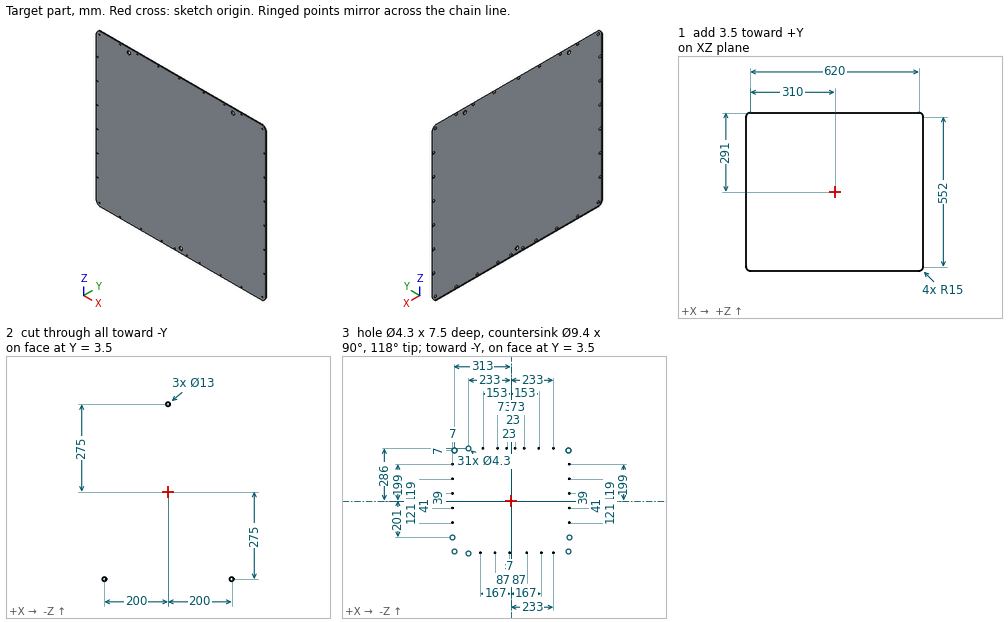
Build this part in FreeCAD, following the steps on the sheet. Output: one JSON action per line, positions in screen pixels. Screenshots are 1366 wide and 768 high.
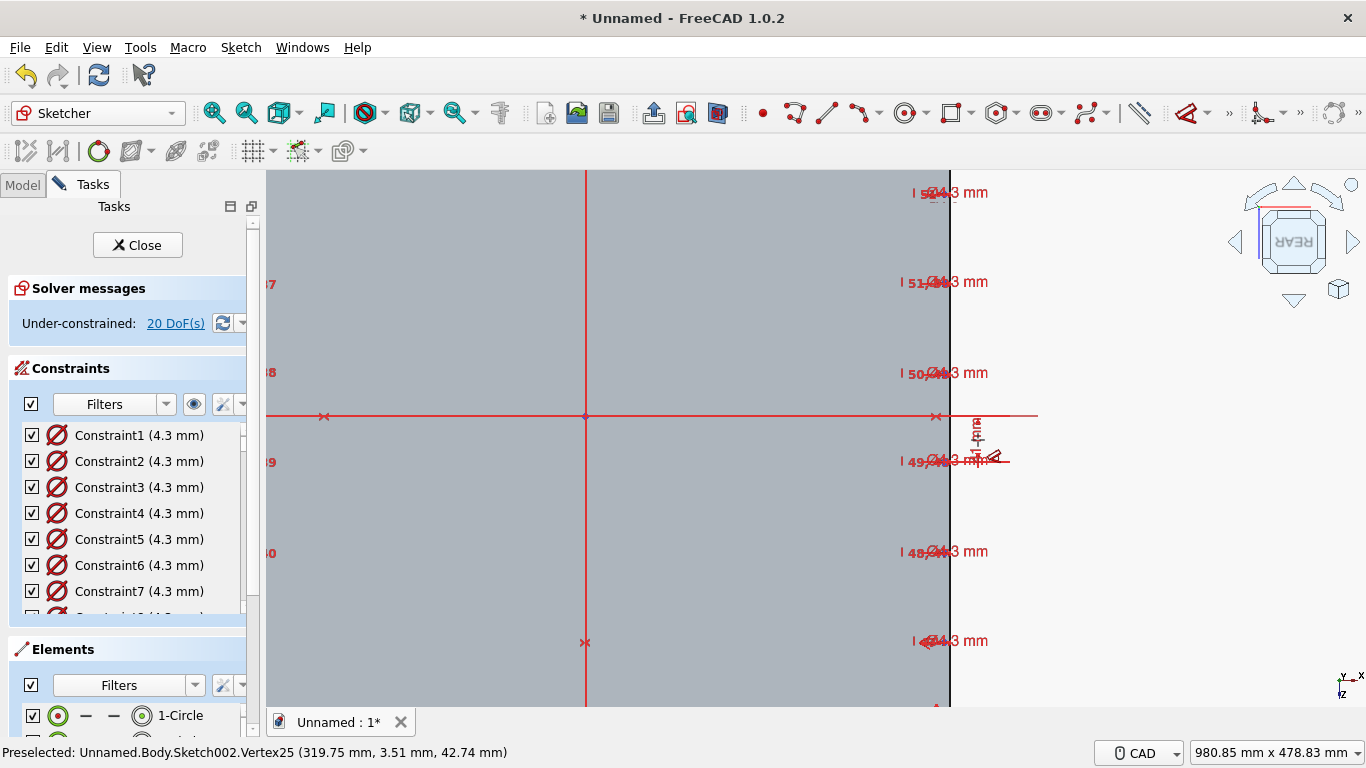
{"action": "left_click", "coordinate": [944, 375]}
{"action": "left_click", "coordinate": [978, 396]}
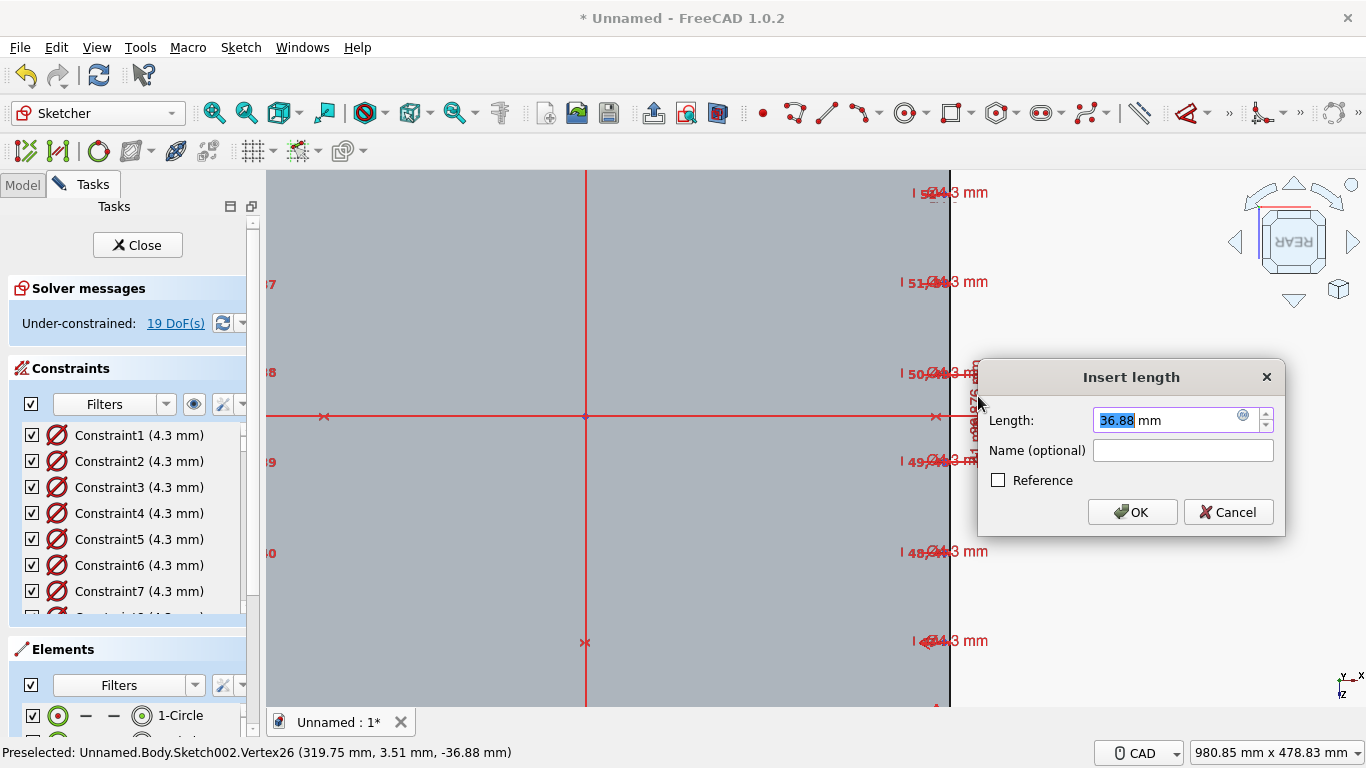
{"action": "type", "text": "39"}
{"action": "key", "text": "Return"}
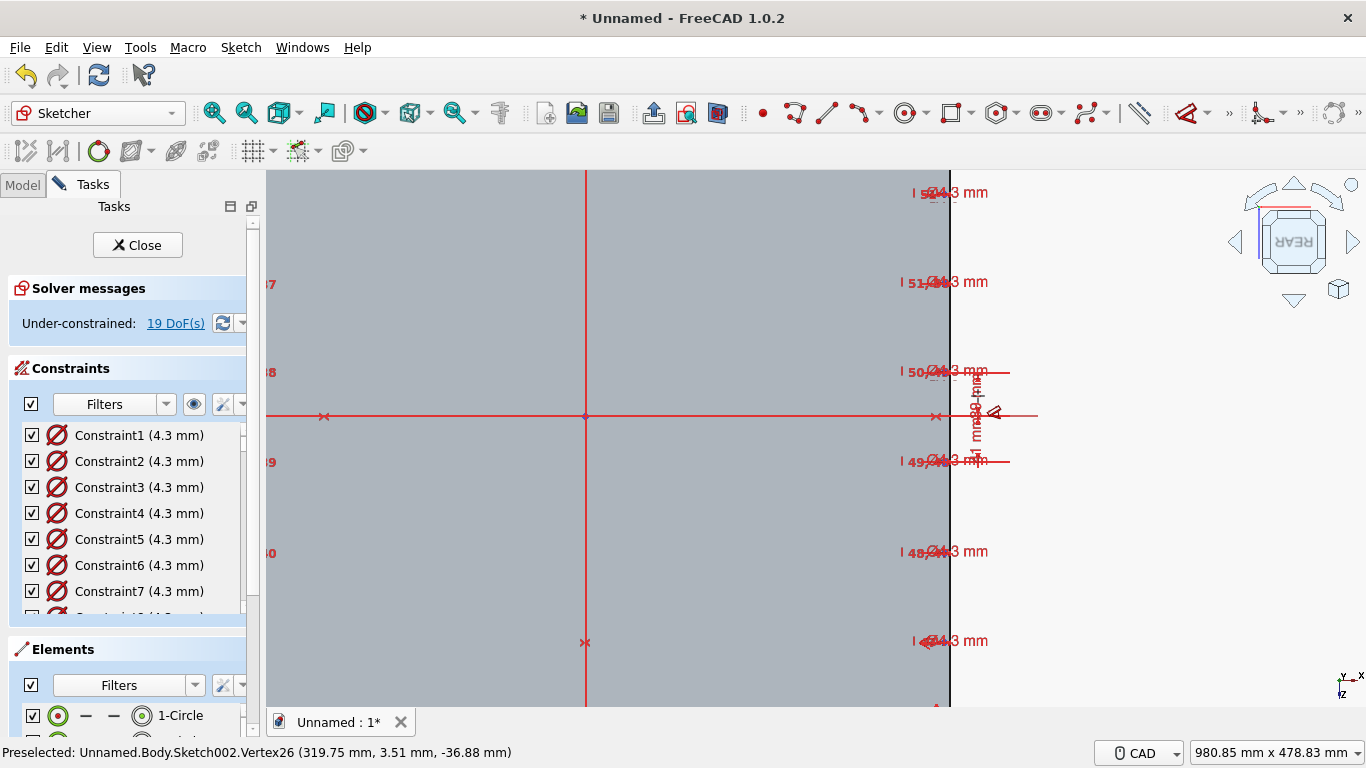
{"action": "scroll", "coordinate": [944, 466], "scroll_direction": "down", "scroll_amount": 3}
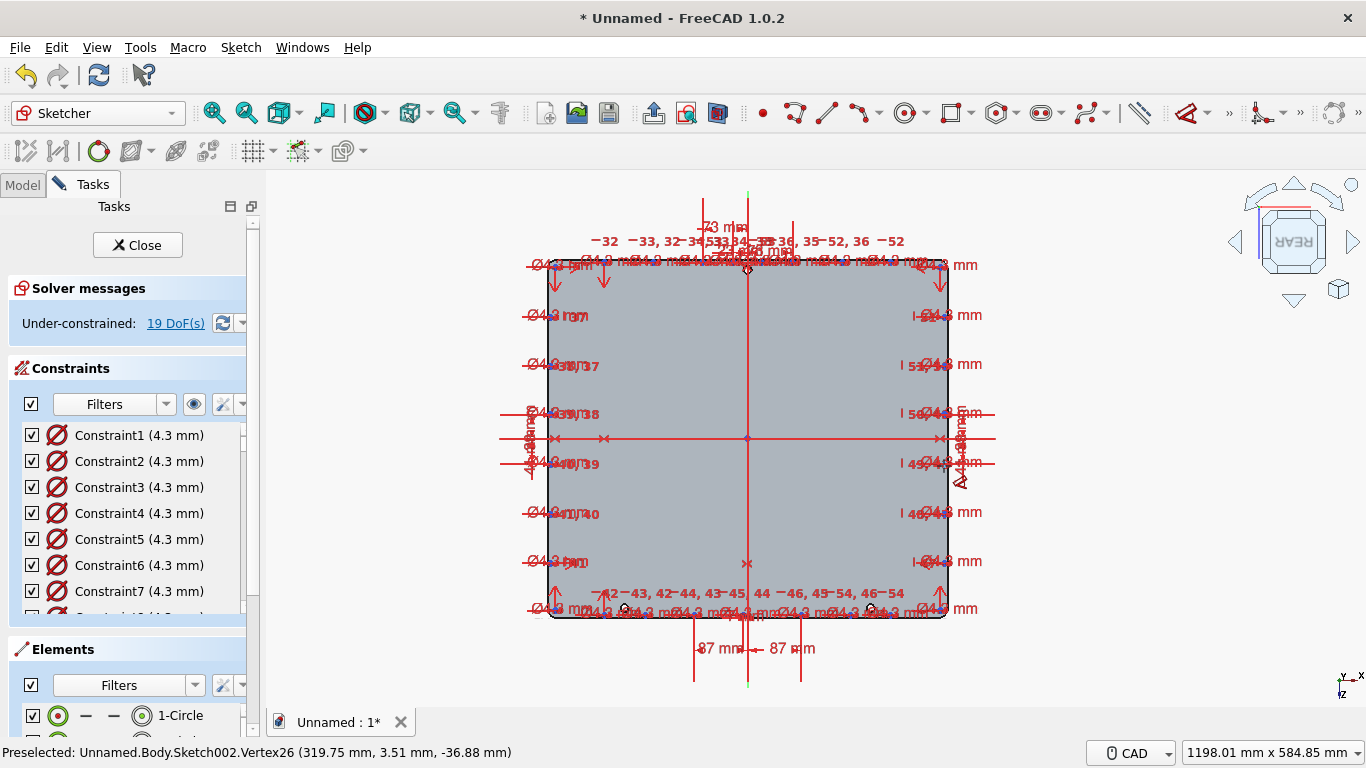
{"action": "scroll", "coordinate": [762, 263], "scroll_direction": "up", "scroll_amount": 6}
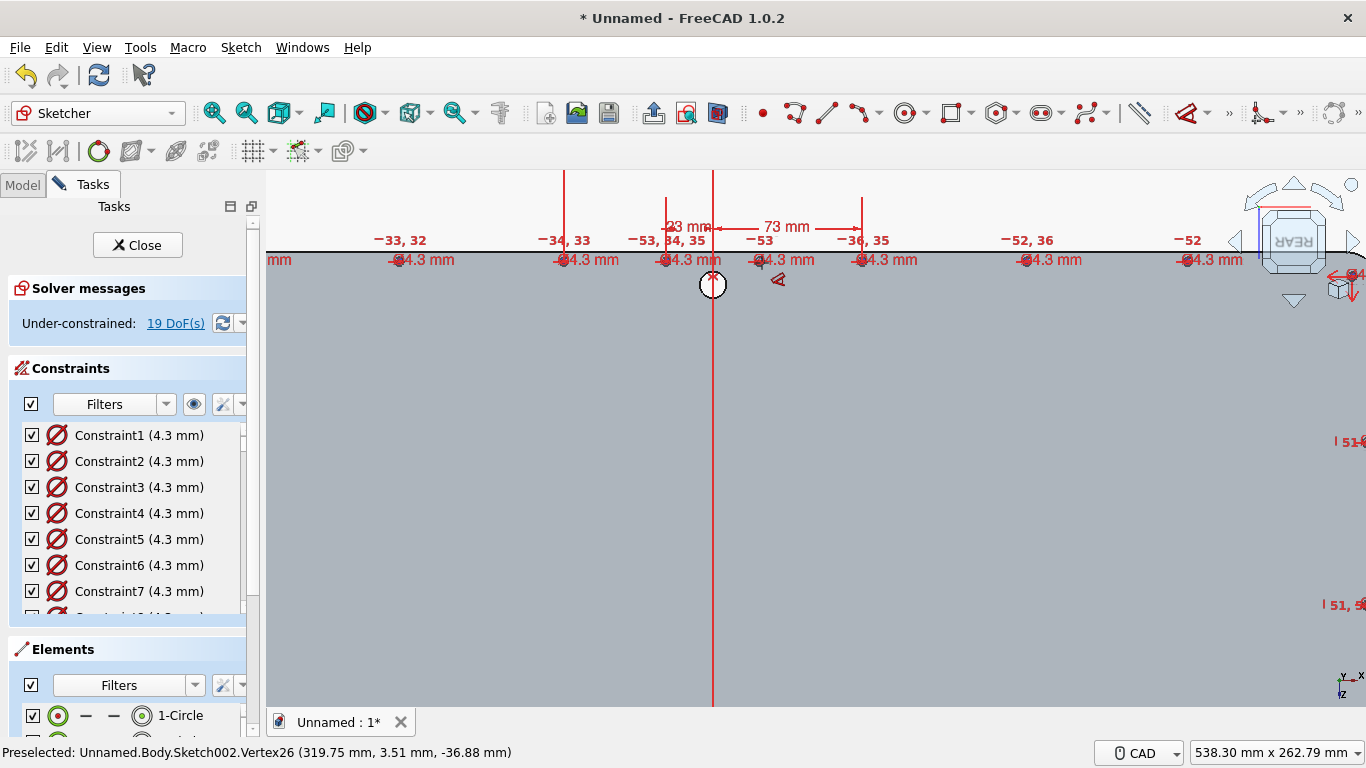
{"action": "left_click", "coordinate": [759, 262]}
{"action": "left_click", "coordinate": [736, 204]}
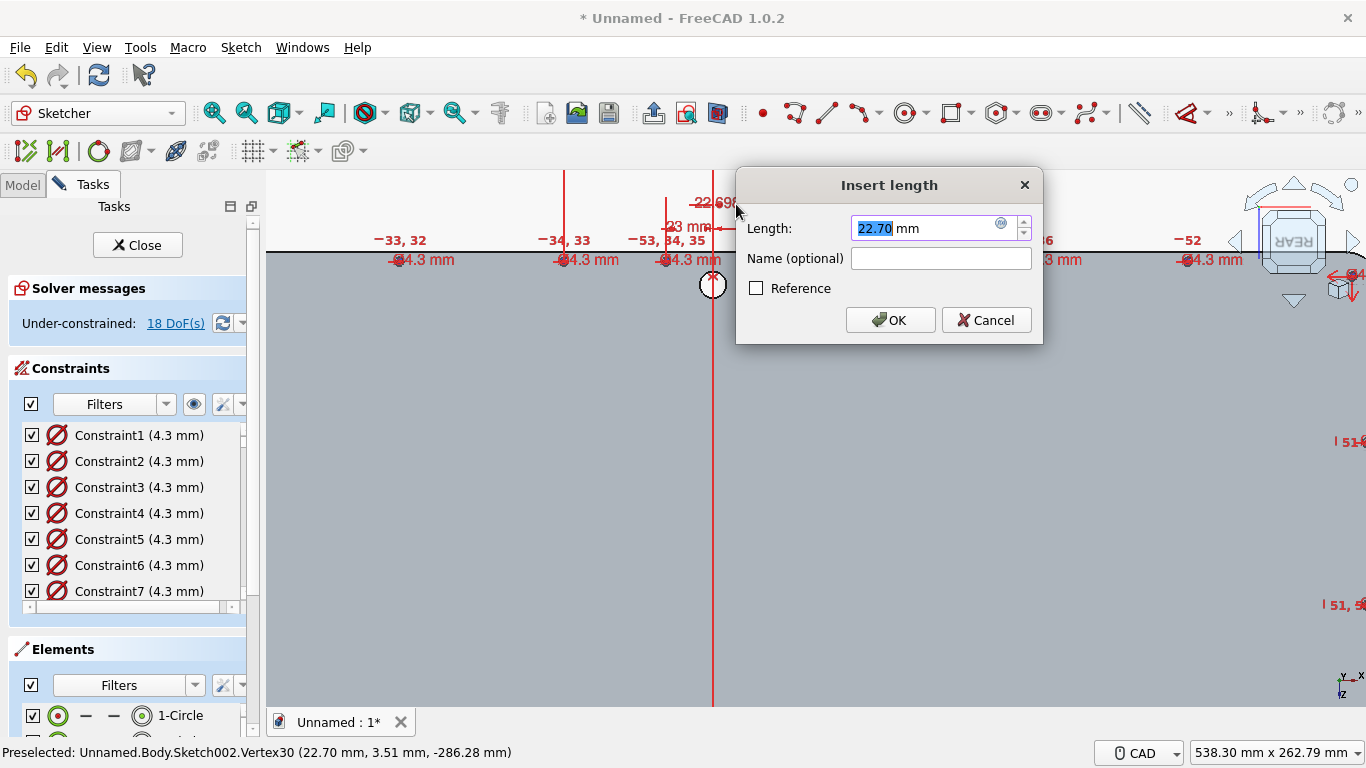
{"action": "type", "text": "23"}
{"action": "key", "text": "Return"}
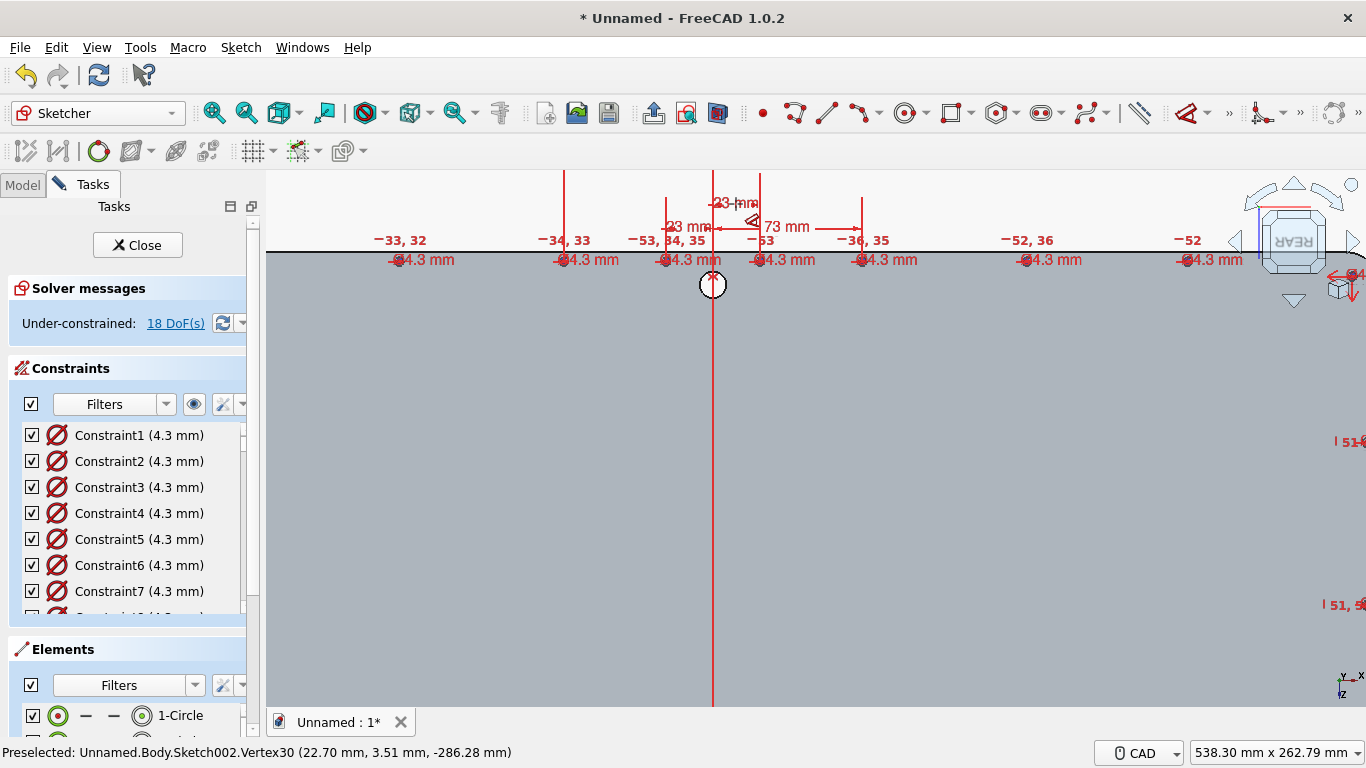
{"action": "scroll", "coordinate": [762, 263], "scroll_direction": "down", "scroll_amount": 6}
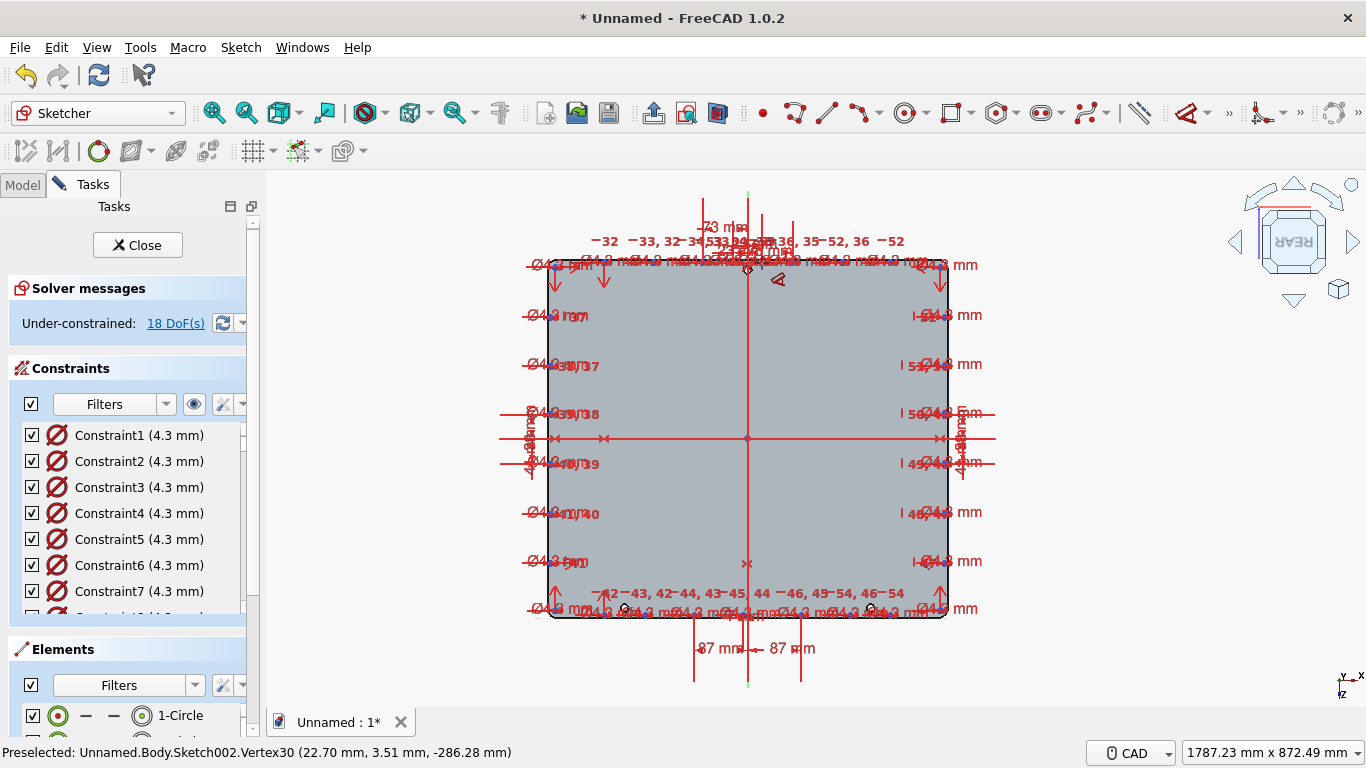
{"action": "scroll", "coordinate": [604, 263], "scroll_direction": "up", "scroll_amount": 12}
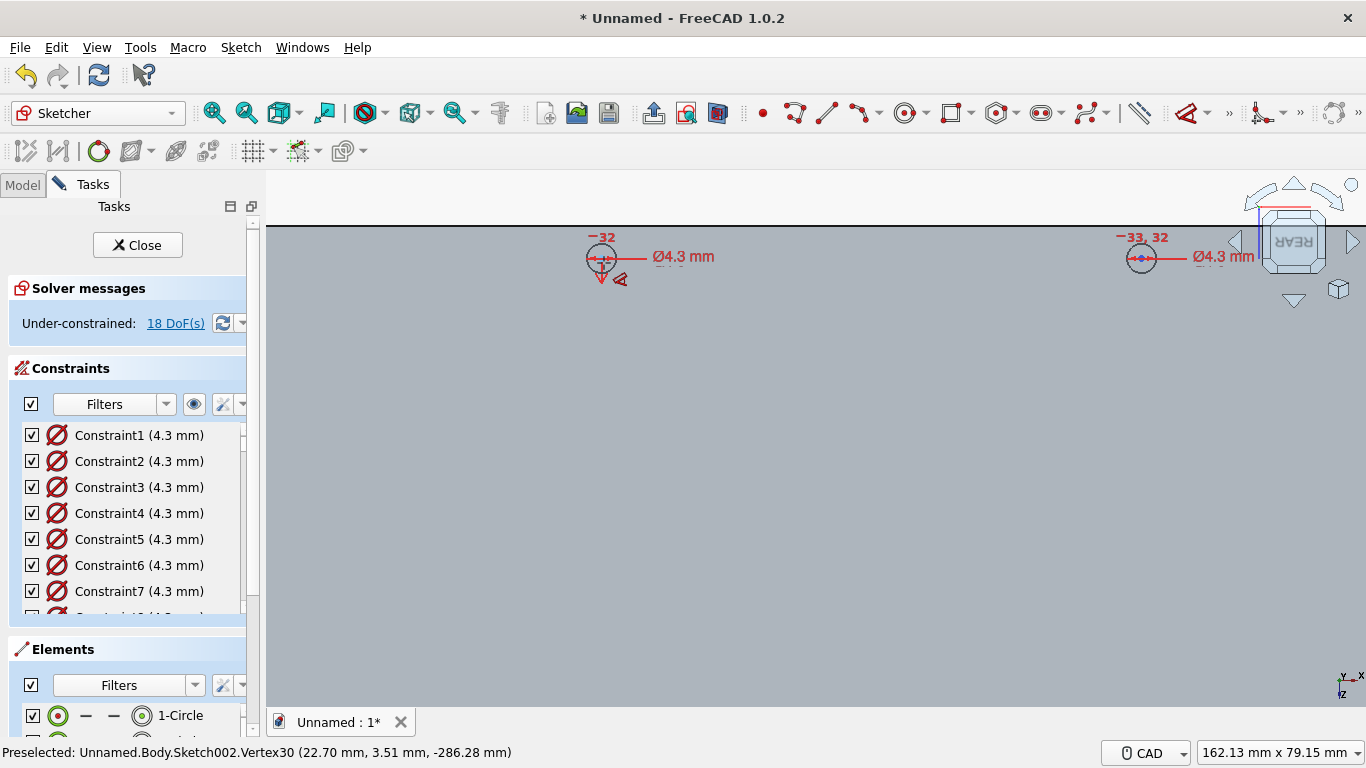
{"action": "left_click", "coordinate": [602, 259]}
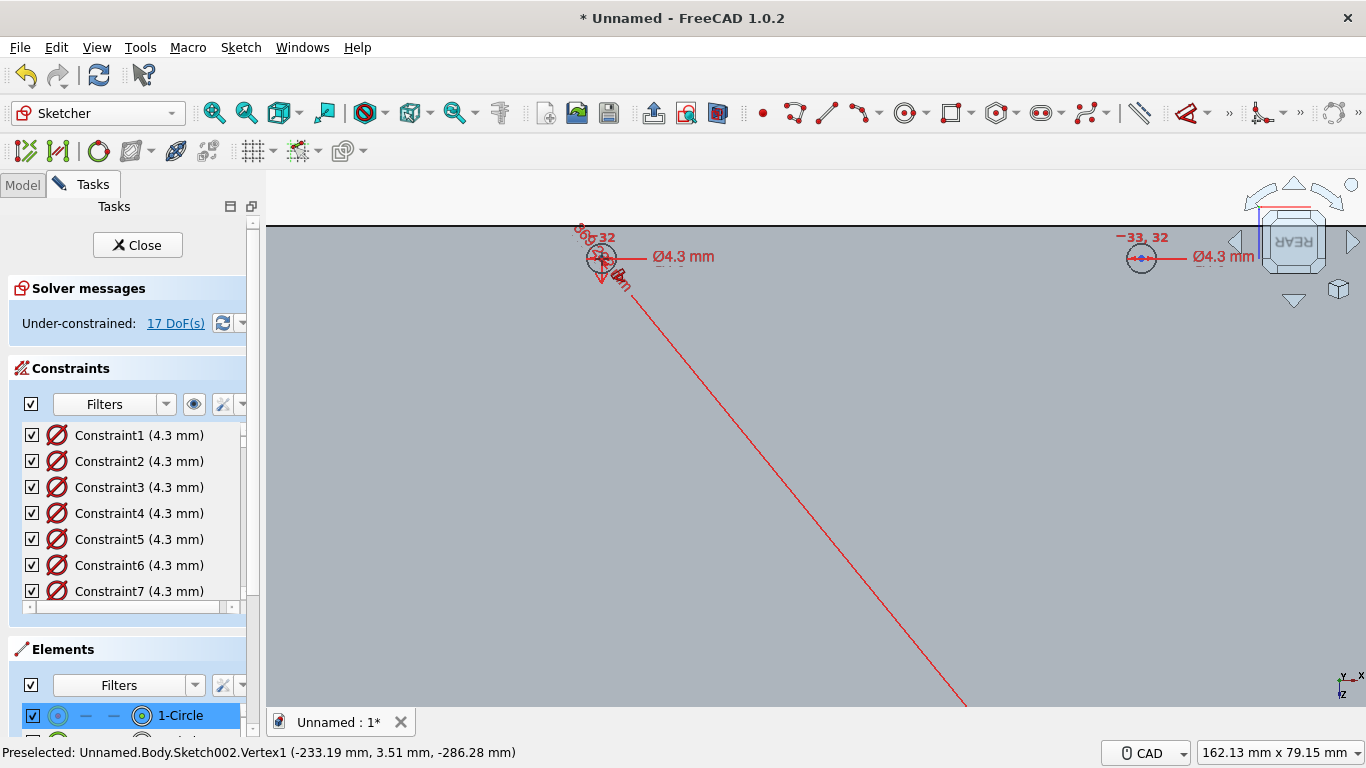
{"action": "scroll", "coordinate": [604, 263], "scroll_direction": "down", "scroll_amount": 12}